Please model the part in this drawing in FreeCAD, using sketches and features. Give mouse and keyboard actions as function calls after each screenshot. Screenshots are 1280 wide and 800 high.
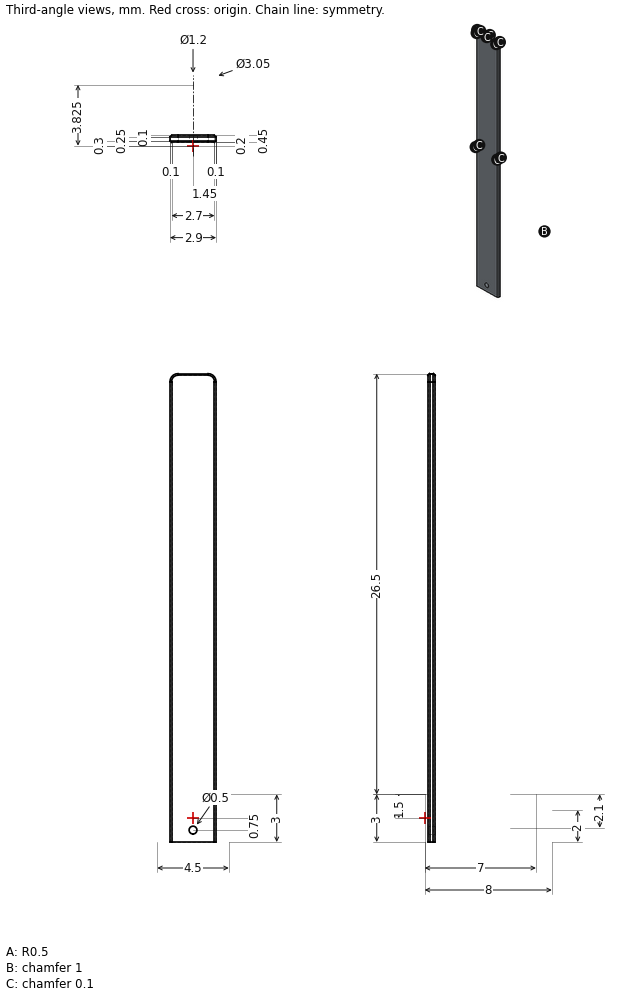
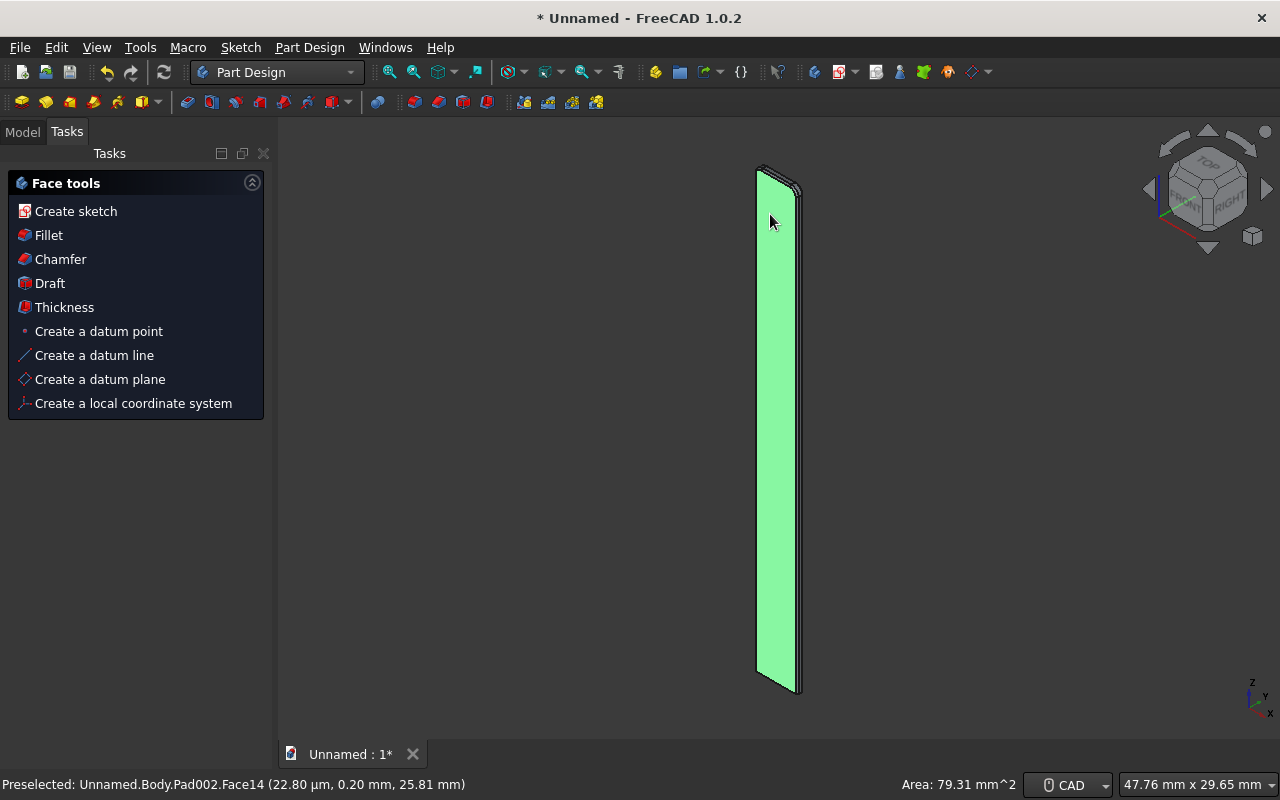
click(840, 72)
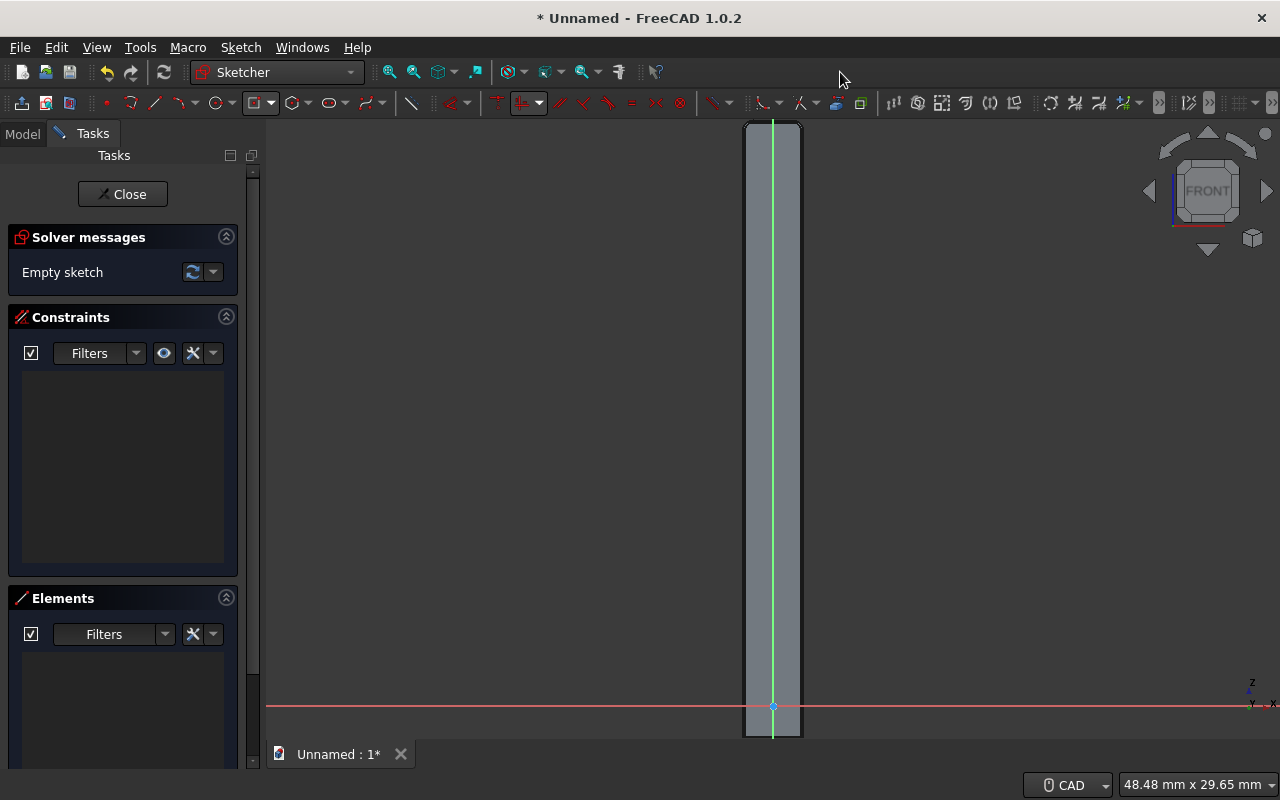
scroll(704, 429, down, 5)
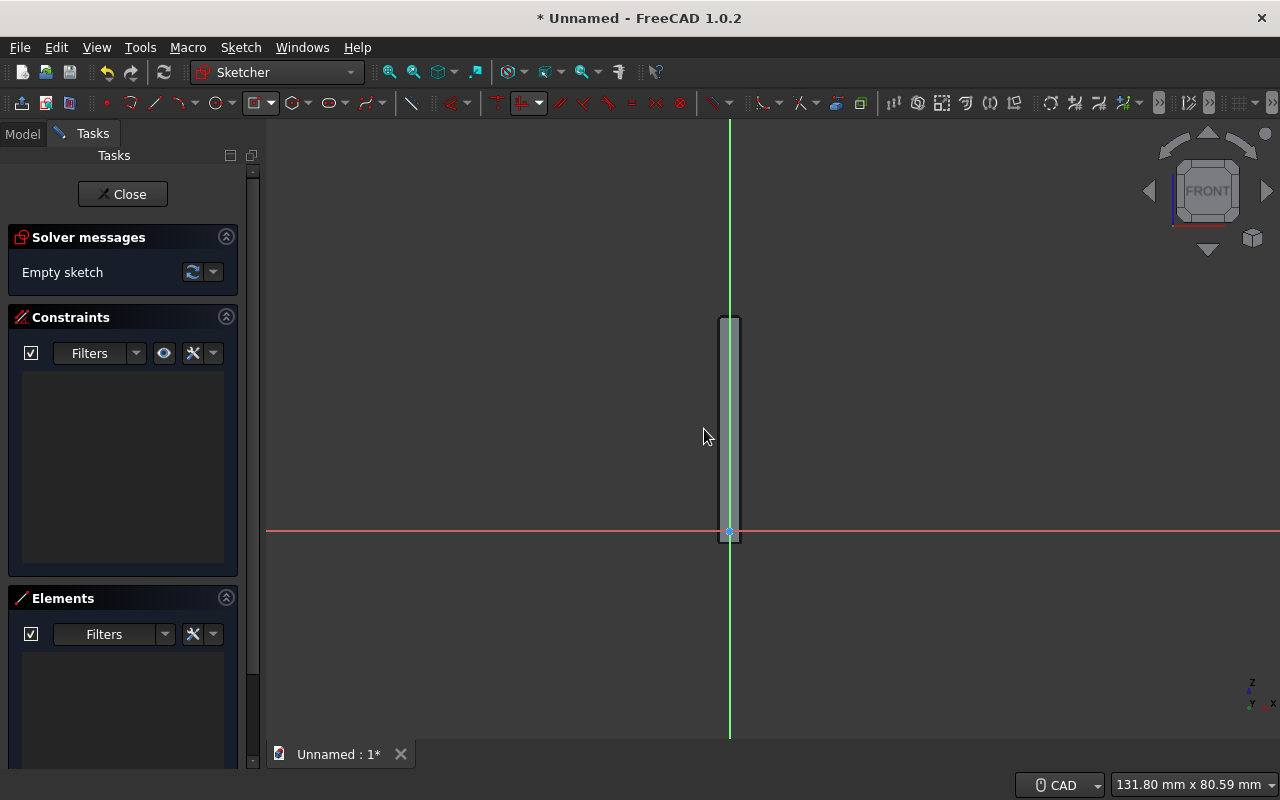
scroll(731, 541, up, 15)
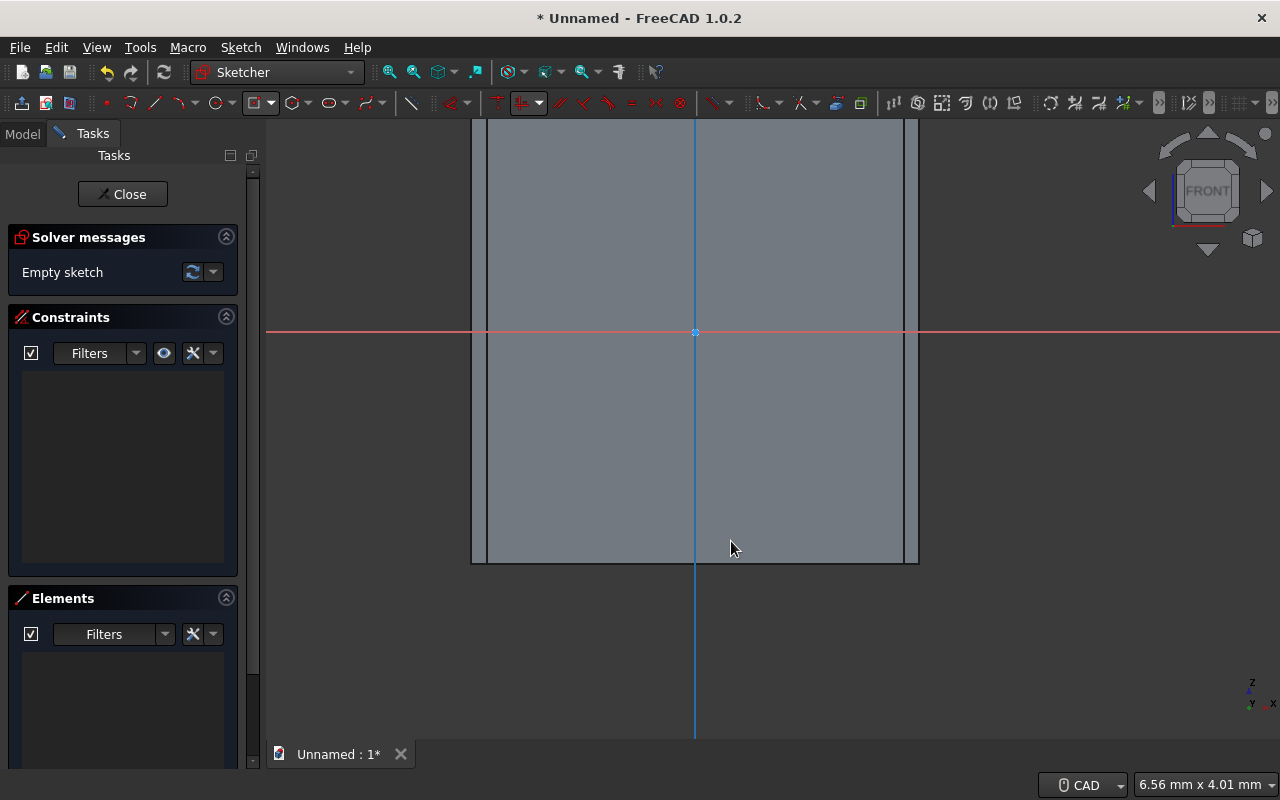
scroll(690, 398, up, 5)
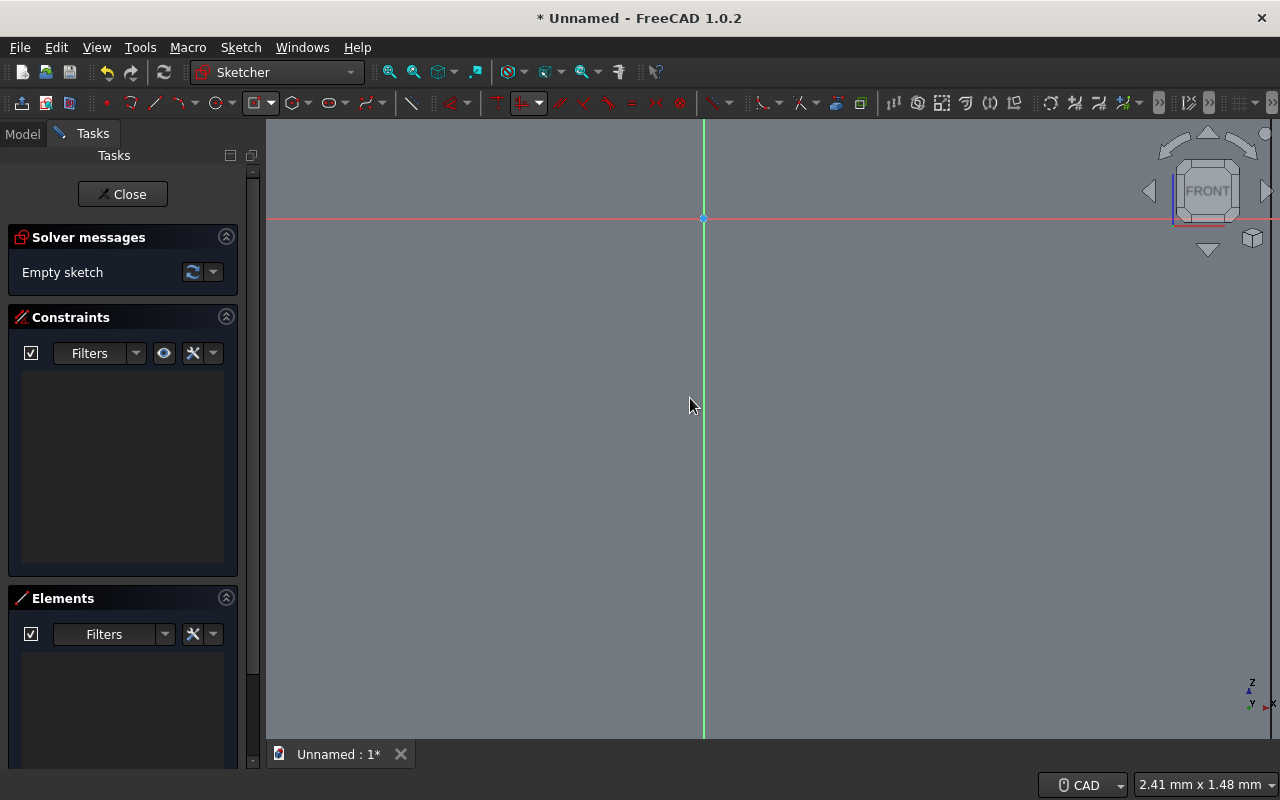
key(g)
key(c)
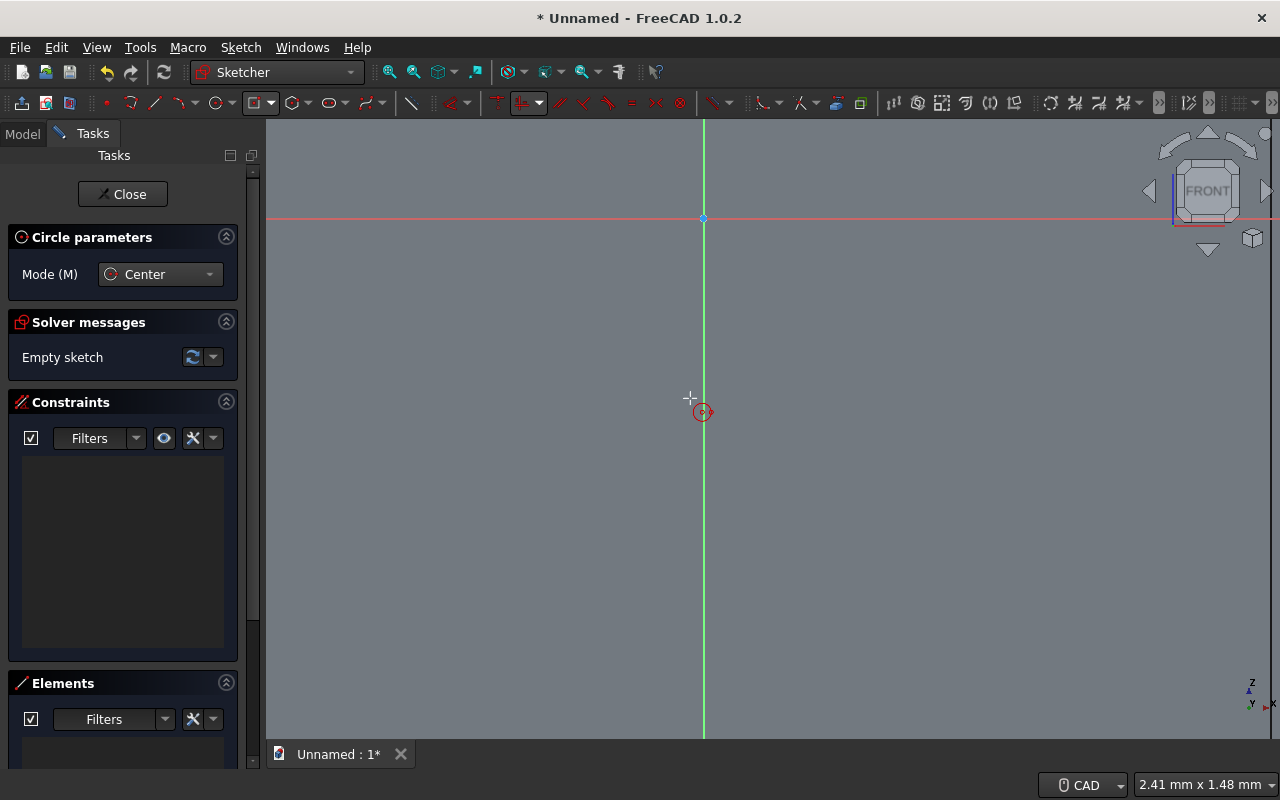
click(704, 534)
click(778, 459)
key(Escape)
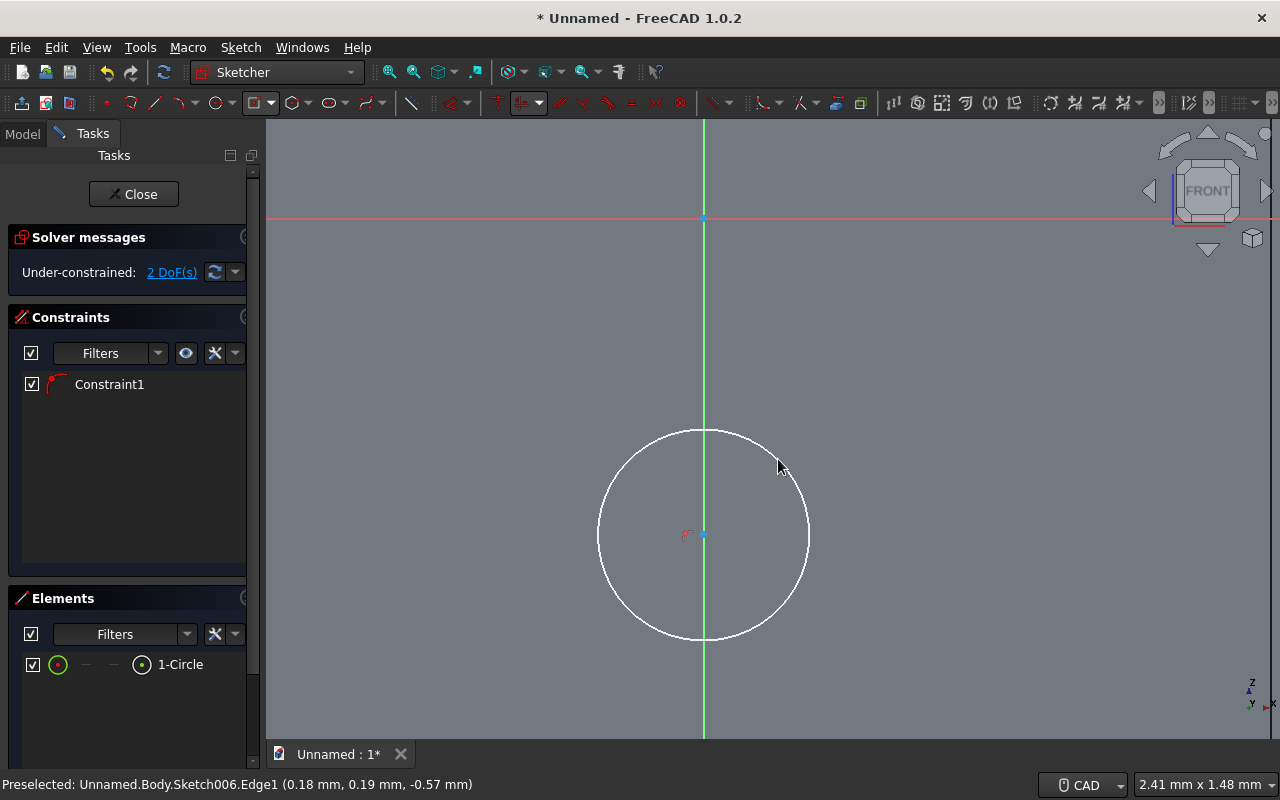
key(d)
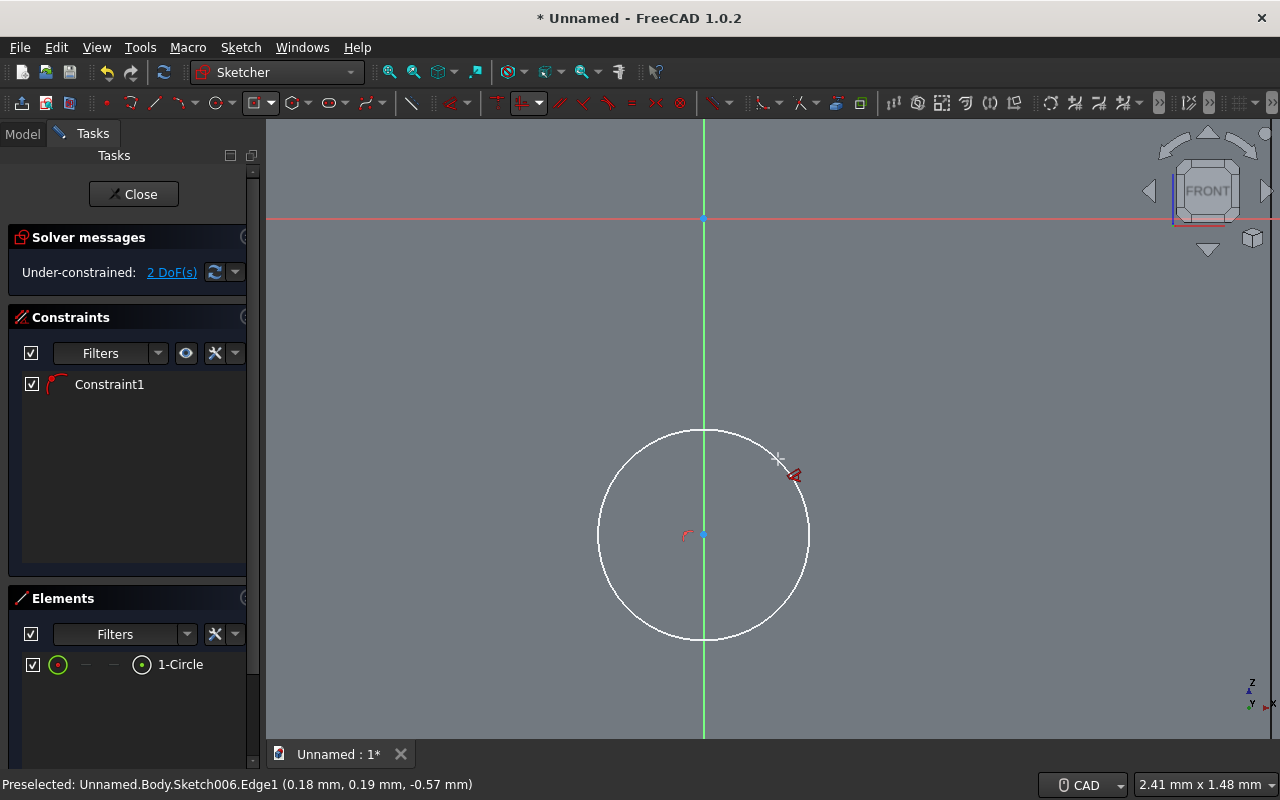
click(778, 460)
click(801, 437)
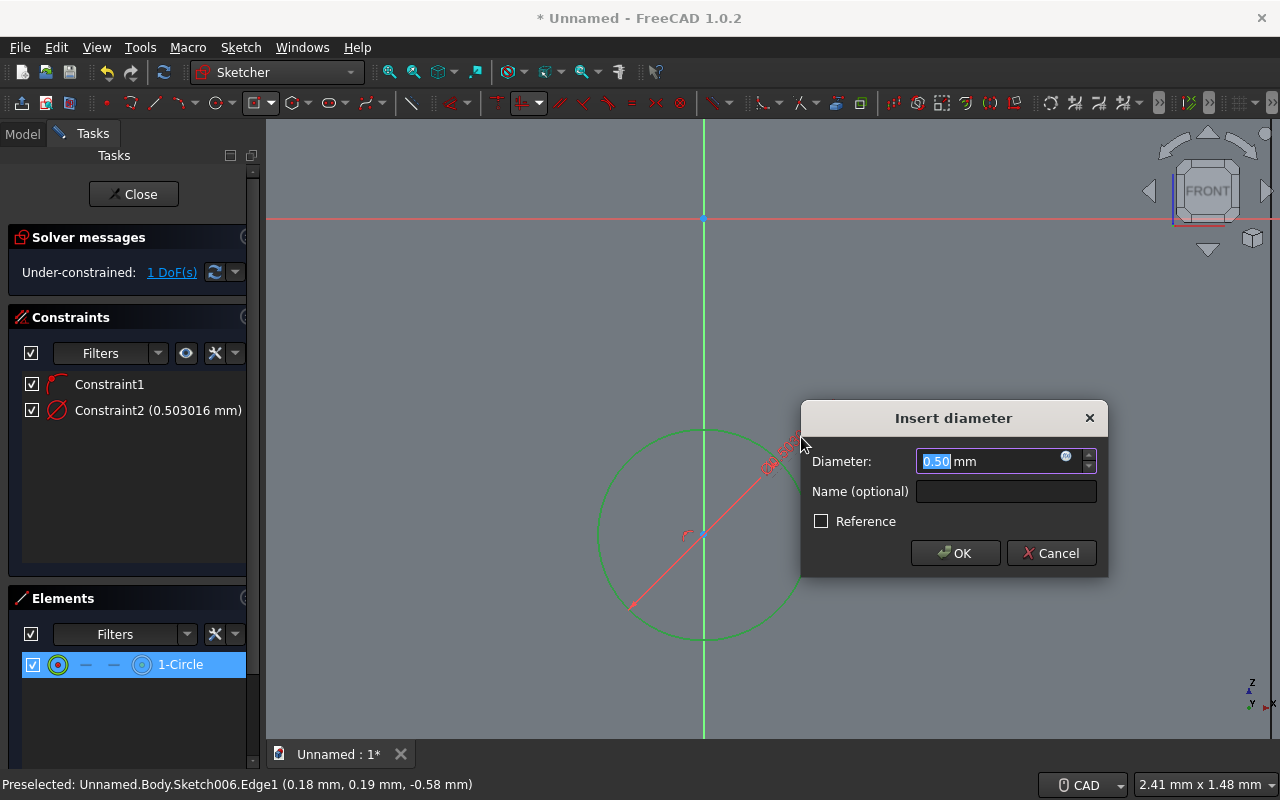
text(0.5)
key(Return)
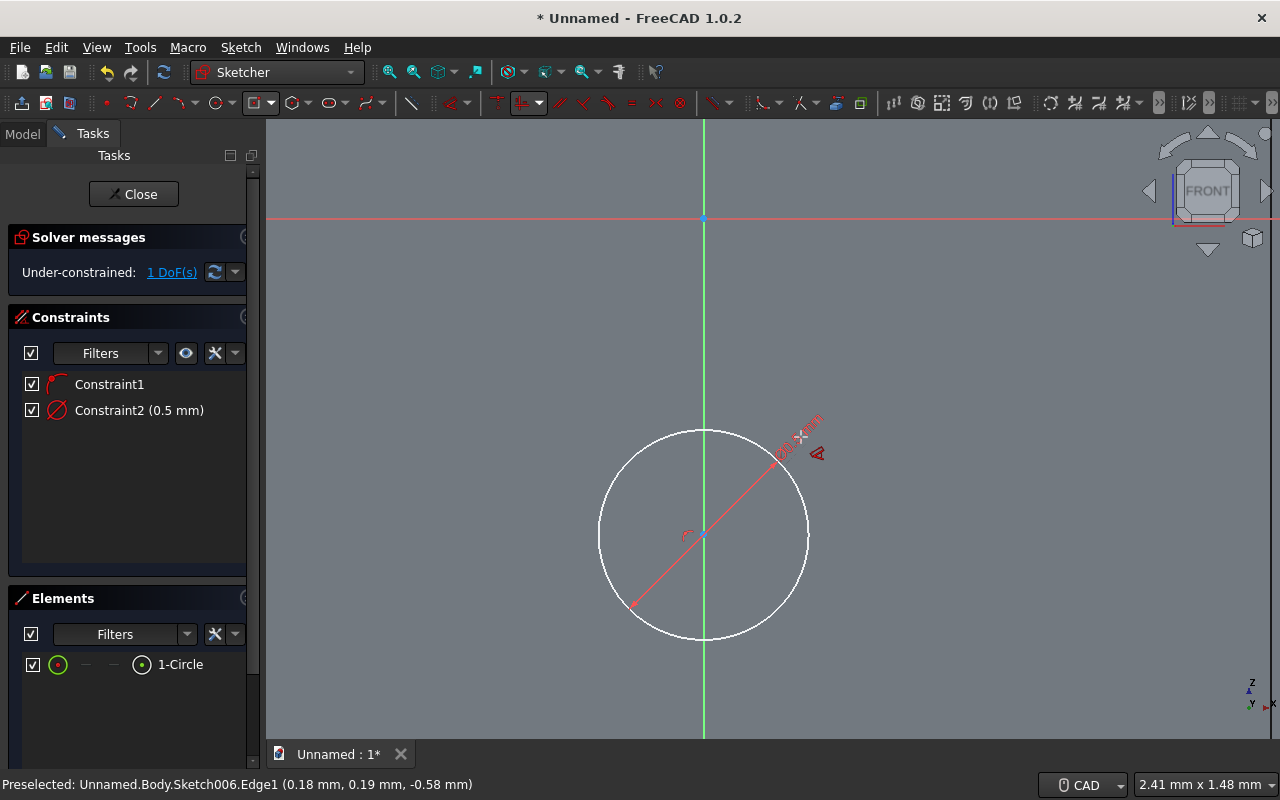
click(704, 535)
click(738, 377)